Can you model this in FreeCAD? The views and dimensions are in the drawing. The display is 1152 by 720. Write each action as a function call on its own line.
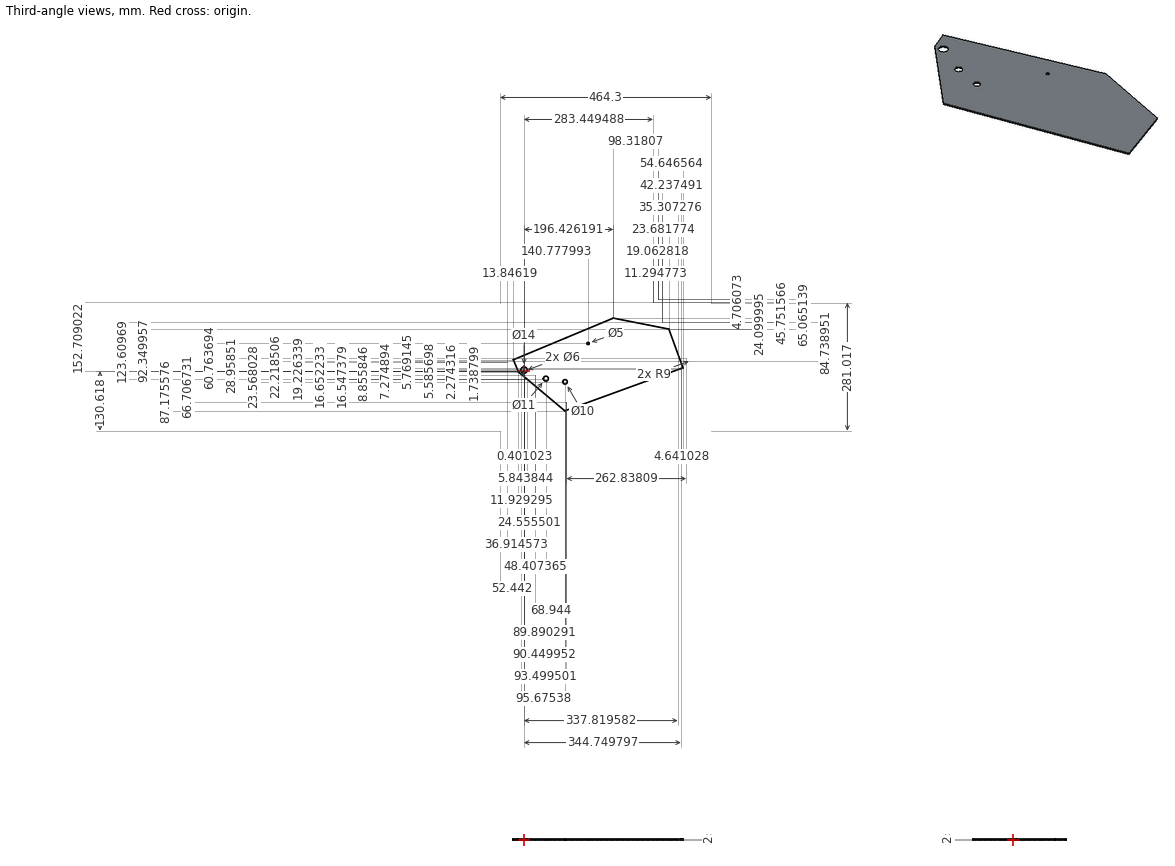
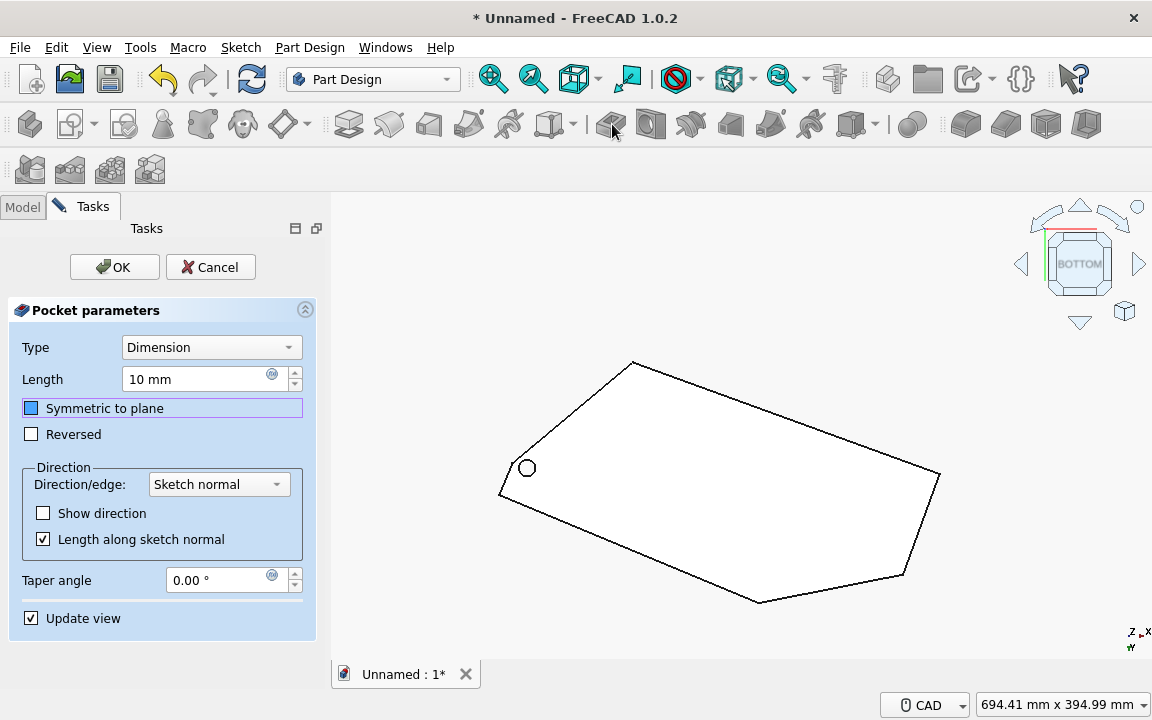
click(115, 267)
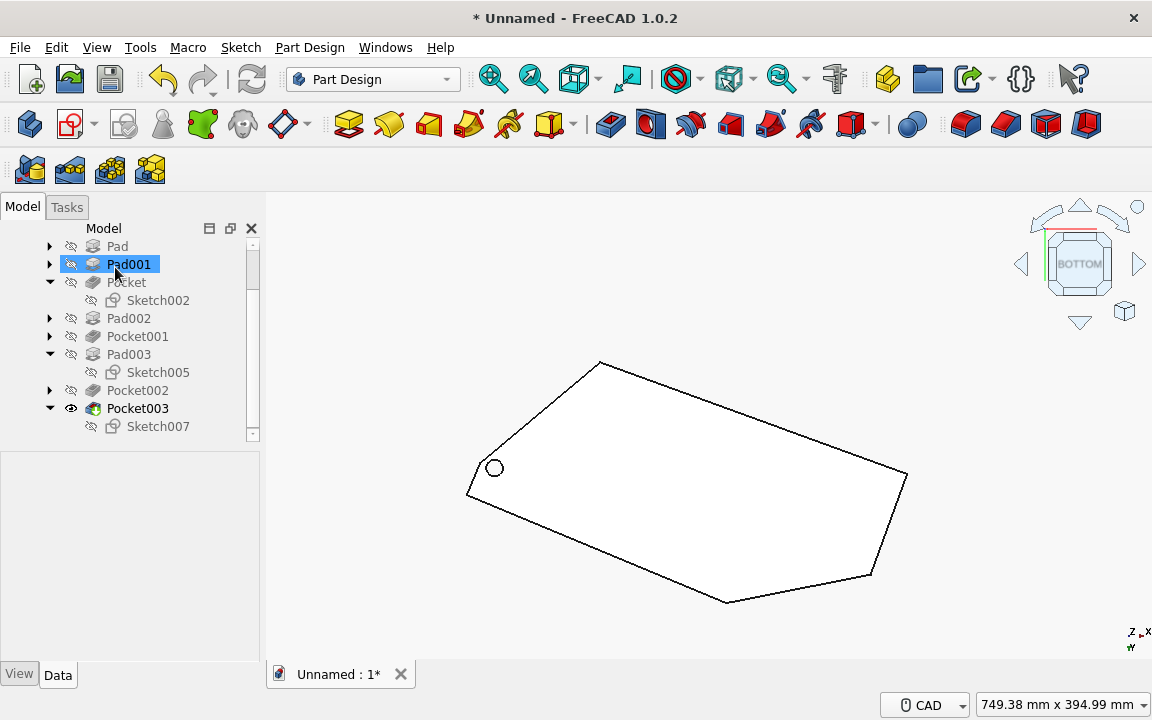
key(0)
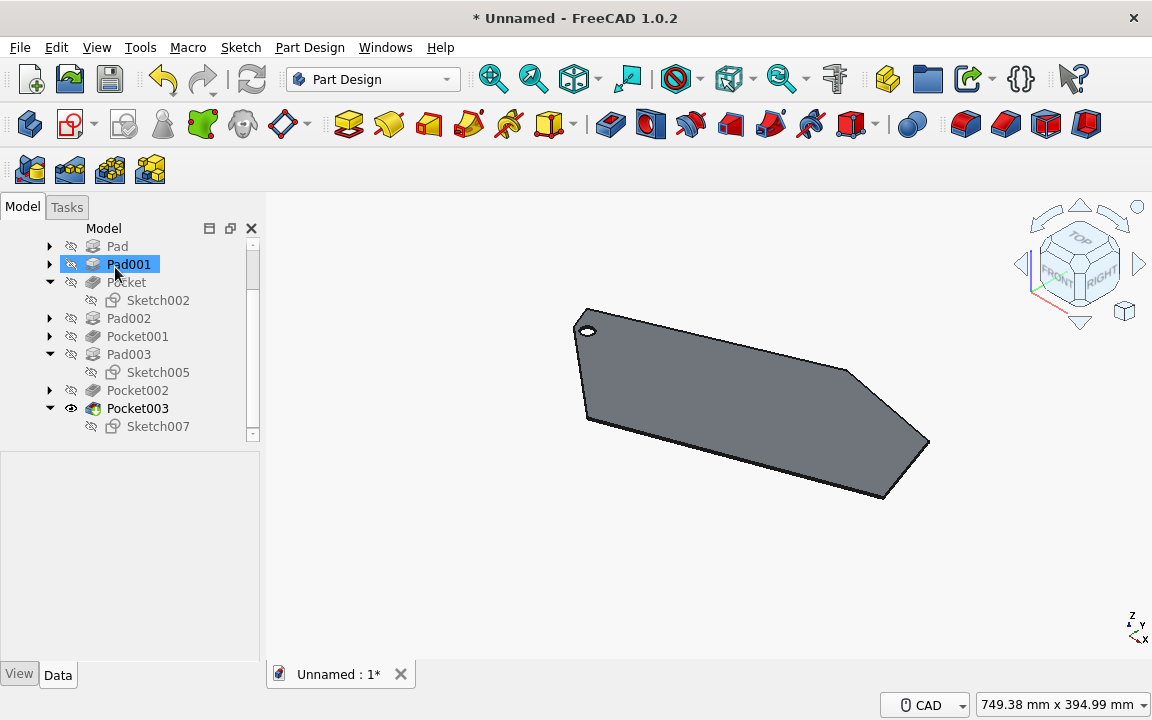
click(734, 403)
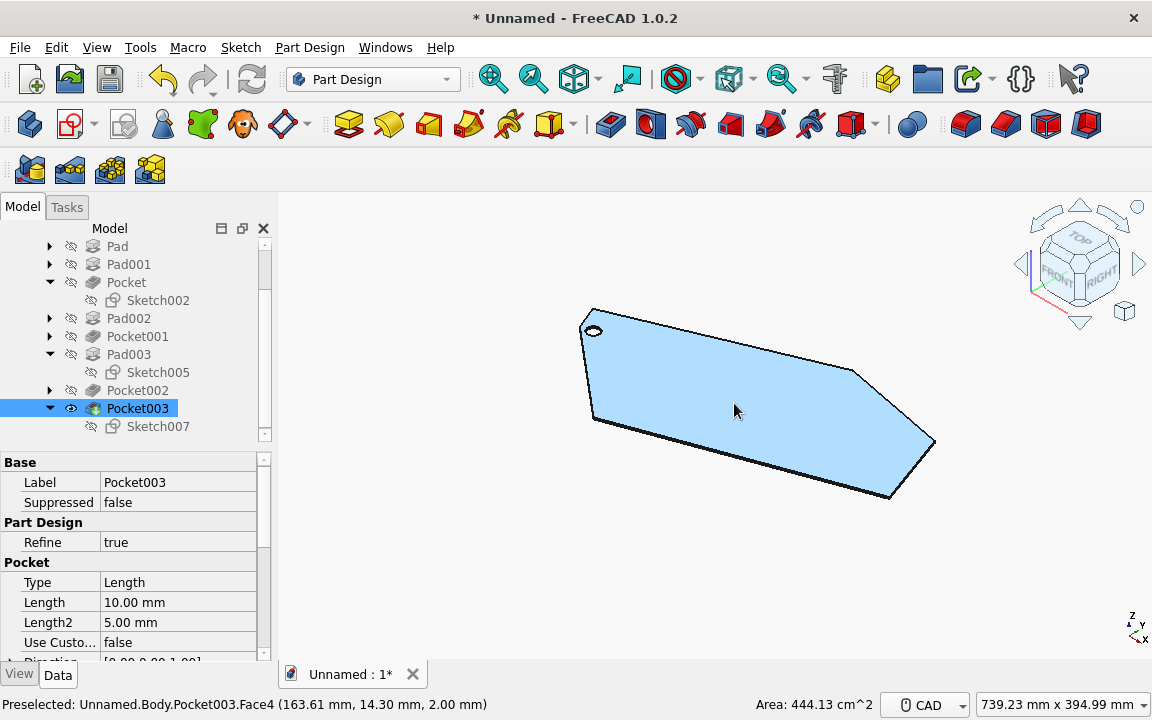
click(70, 124)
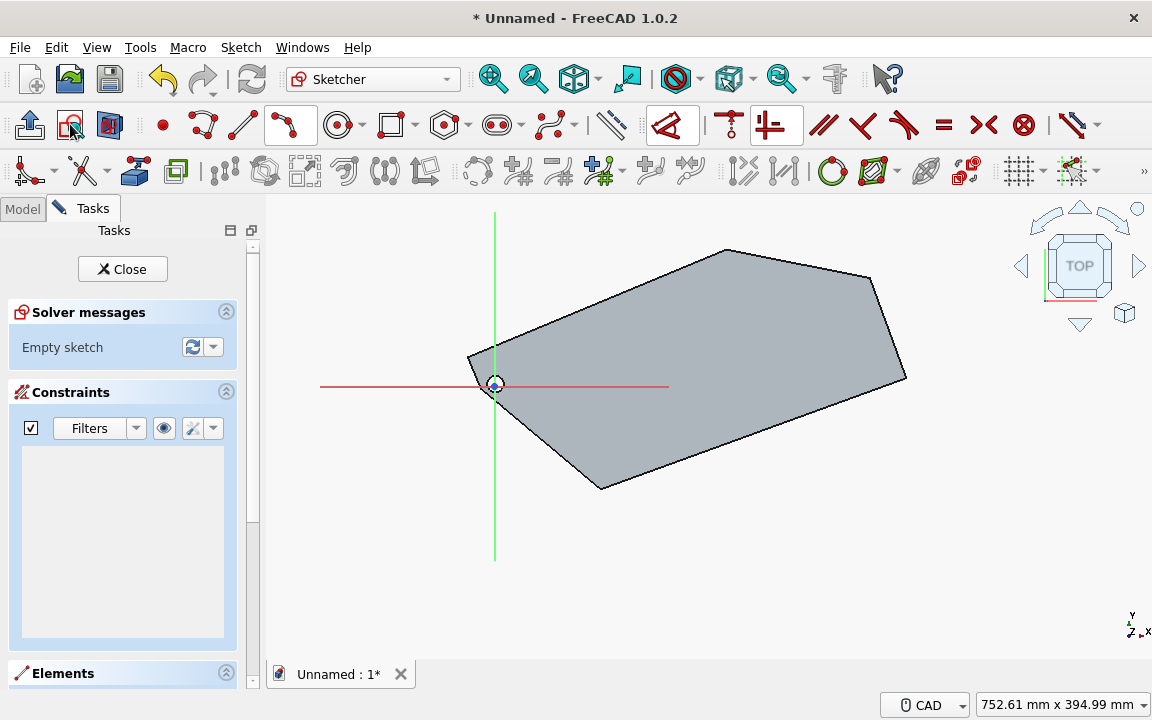
scroll(662, 309, up, 15)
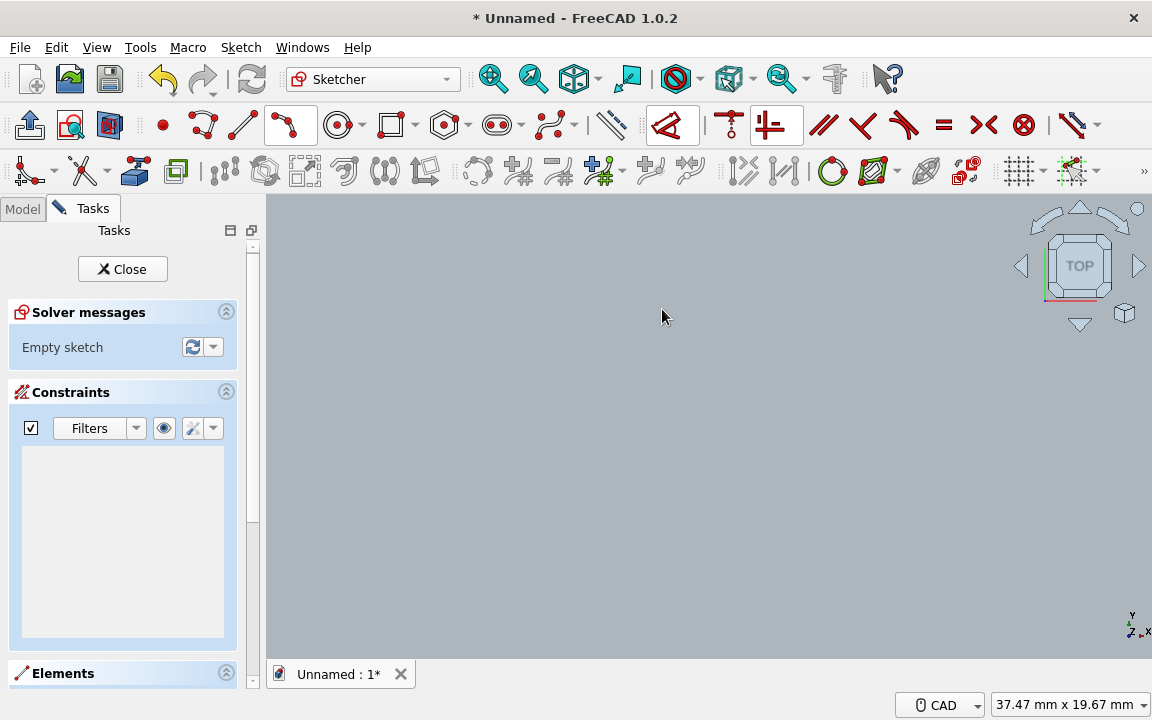
scroll(617, 430, up, 4)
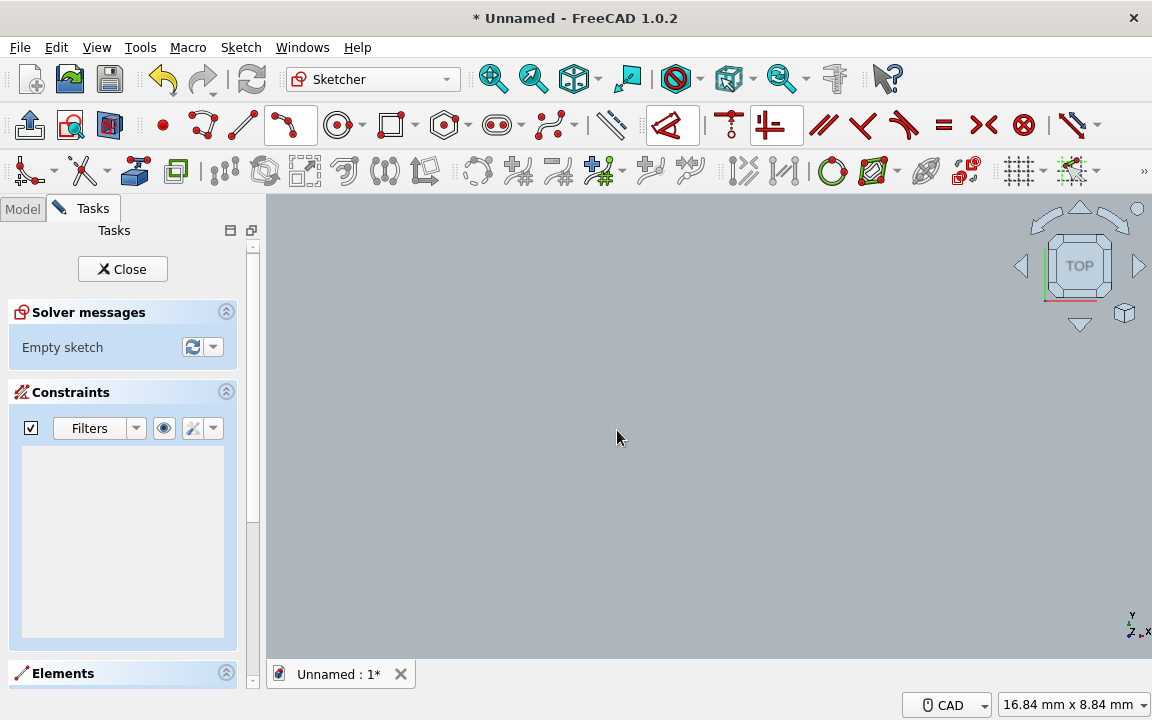
key(g)
key(c)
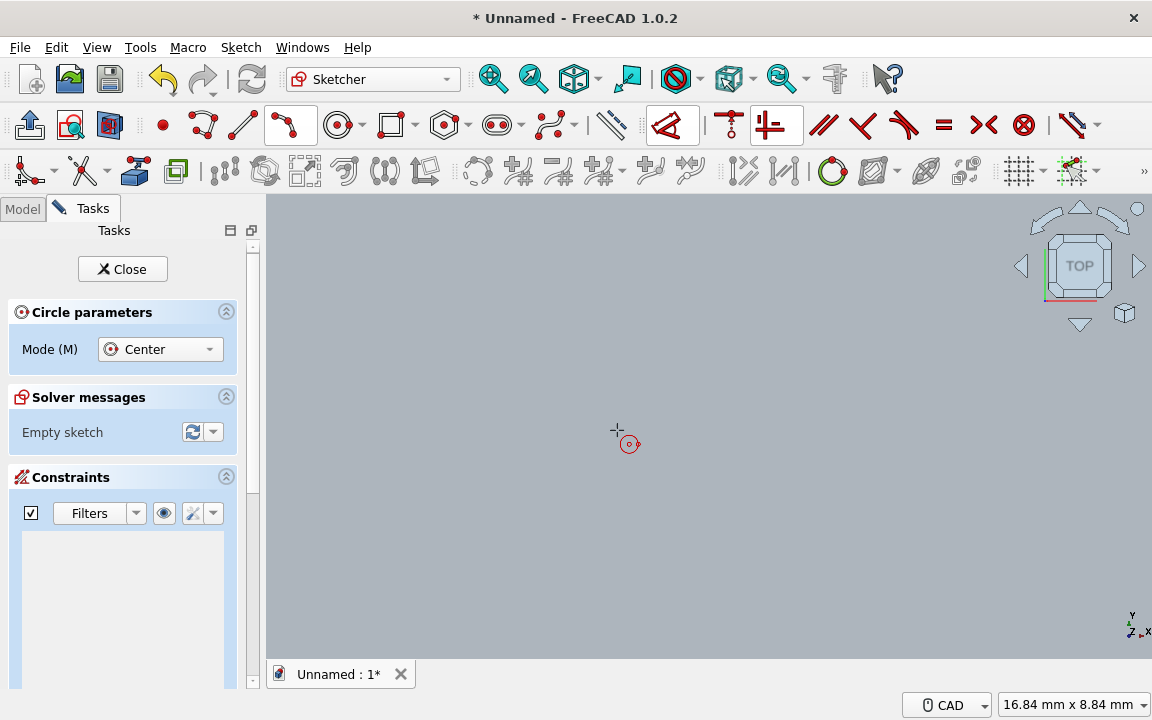
click(640, 426)
move(733, 333)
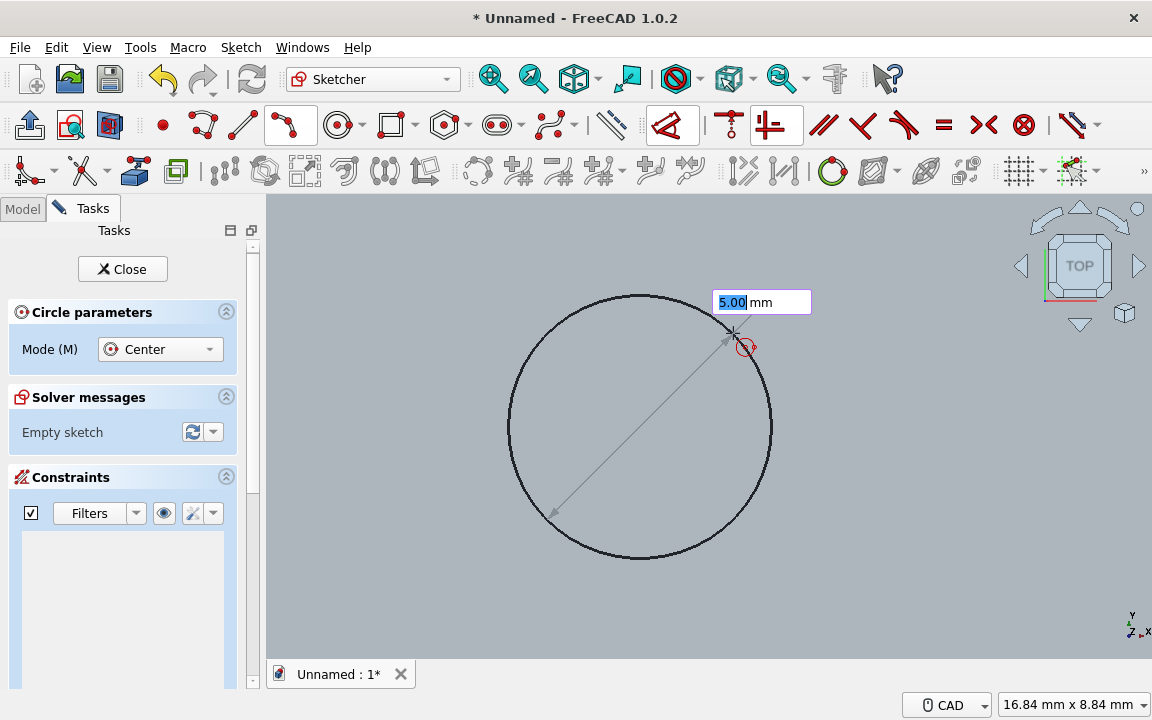
text(5)
key(Return)
key(Escape)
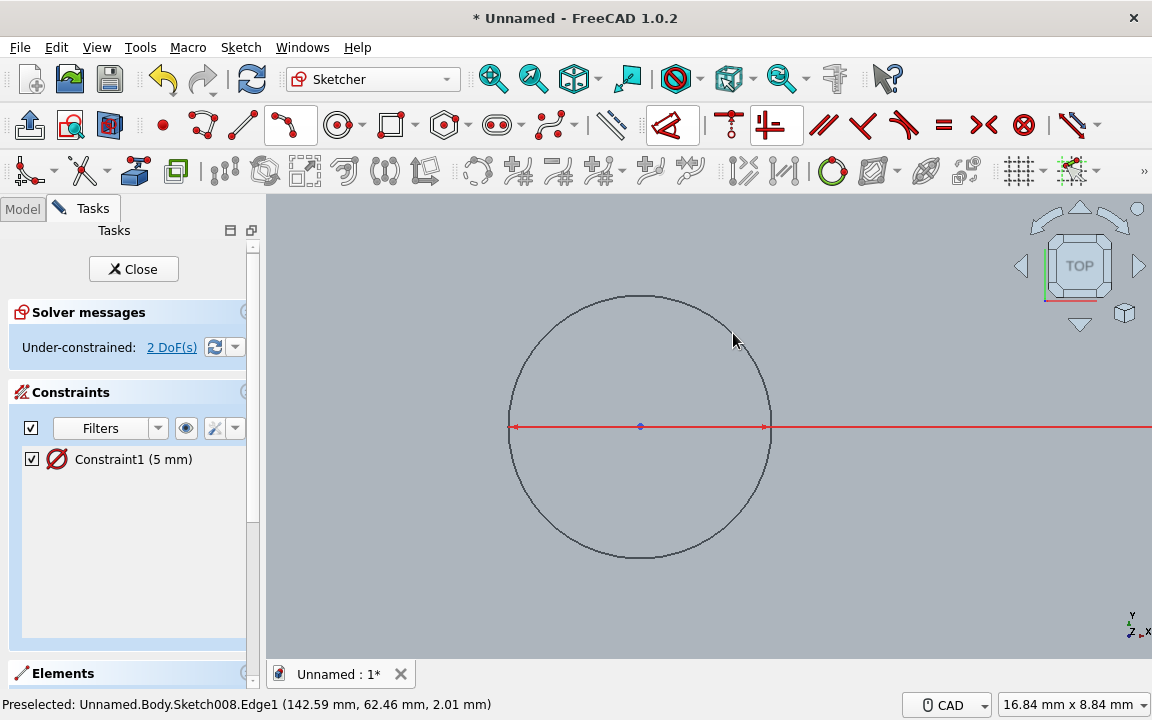
click(640, 427)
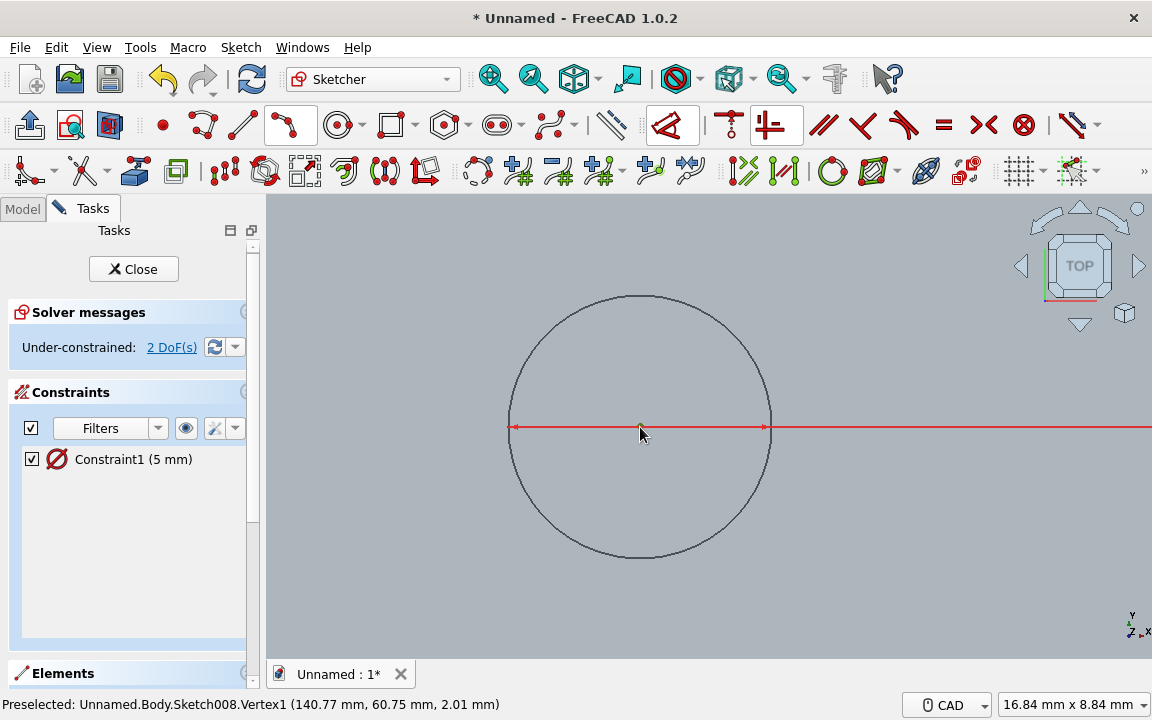
key(i)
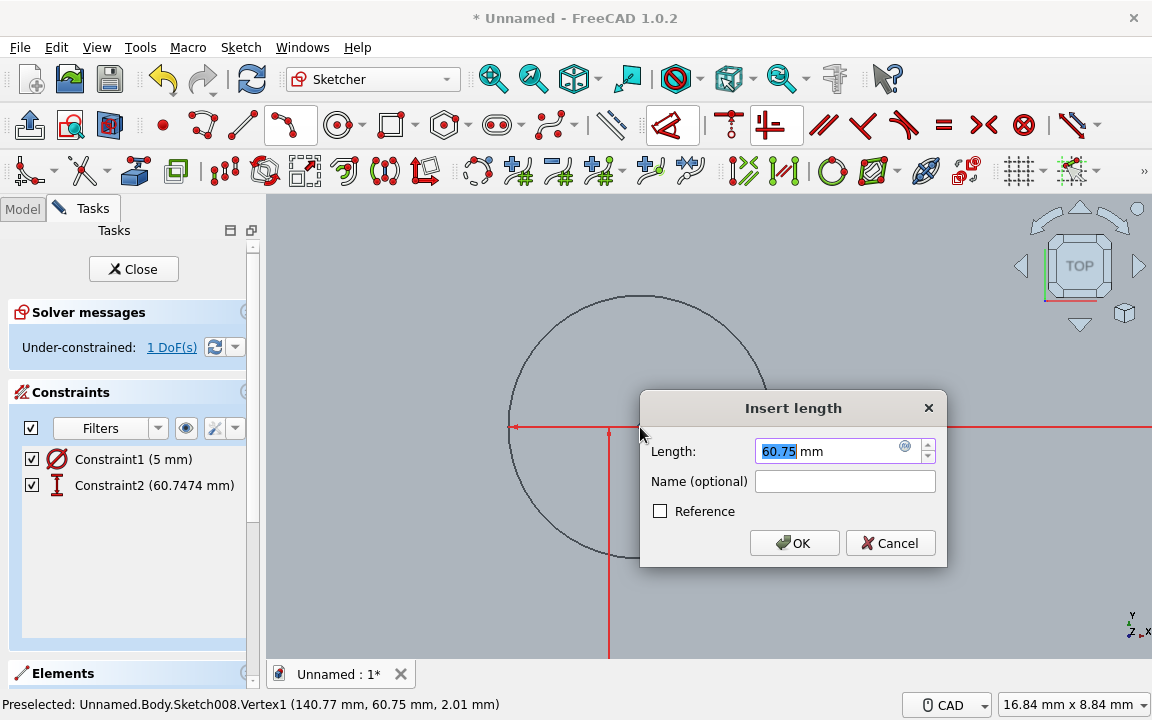
text(60.763694)
key(Return)